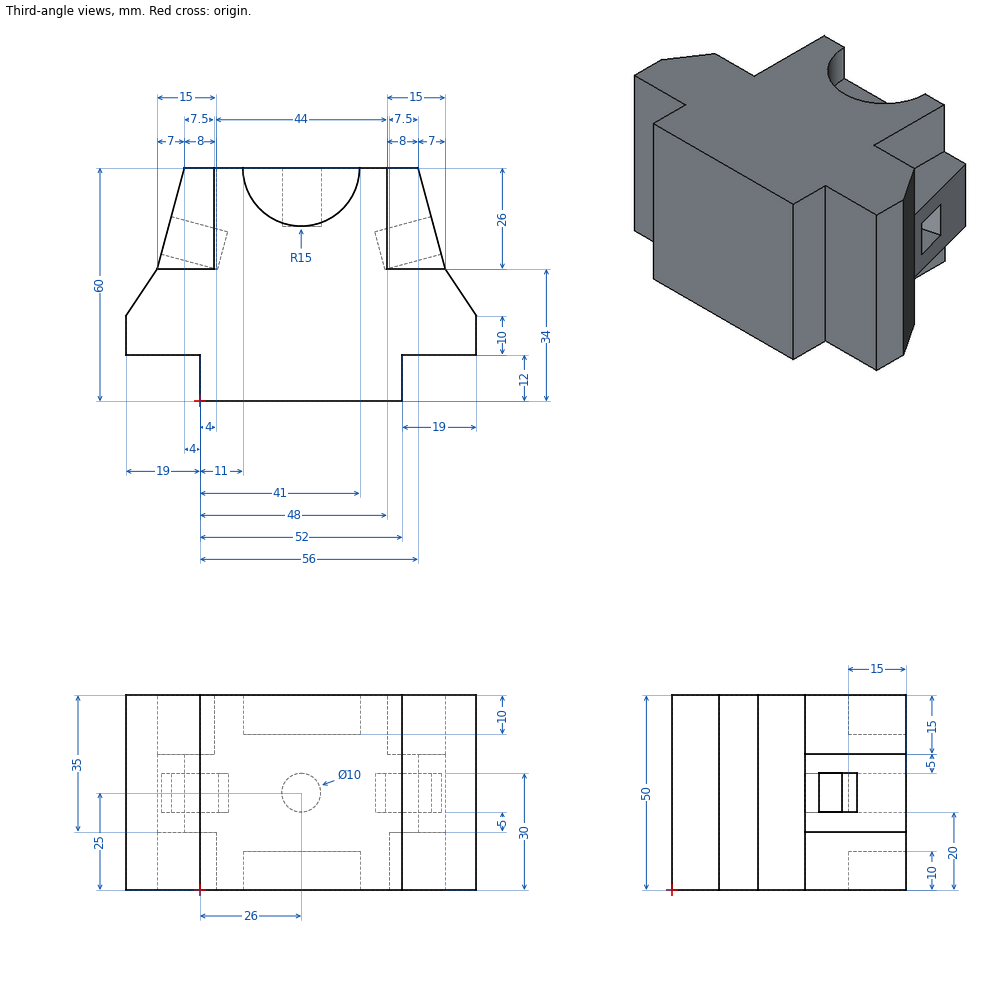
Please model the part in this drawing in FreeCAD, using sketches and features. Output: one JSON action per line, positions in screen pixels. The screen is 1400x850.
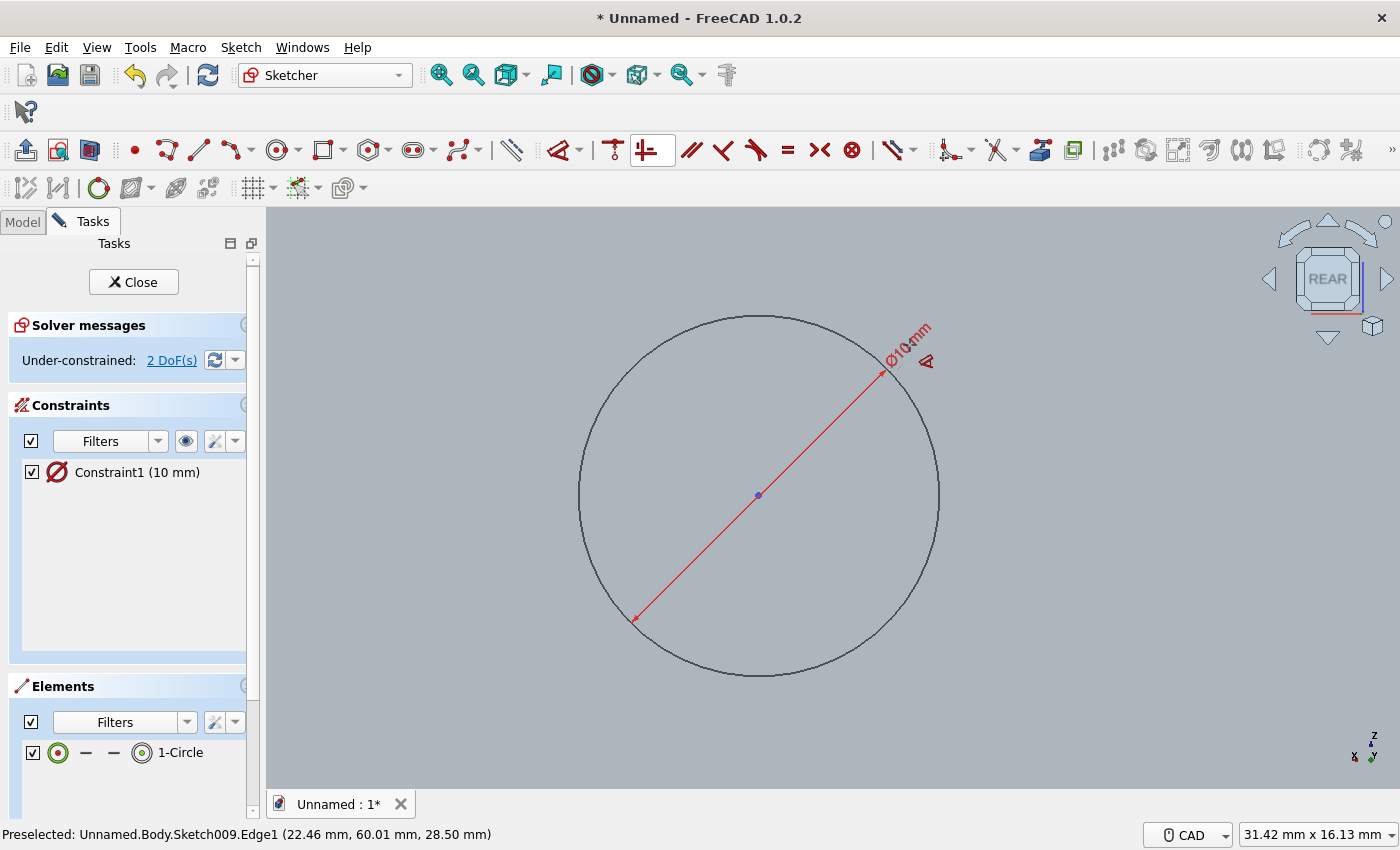
{"action": "left_click", "coordinate": [759, 496]}
{"action": "left_click", "coordinate": [997, 462]}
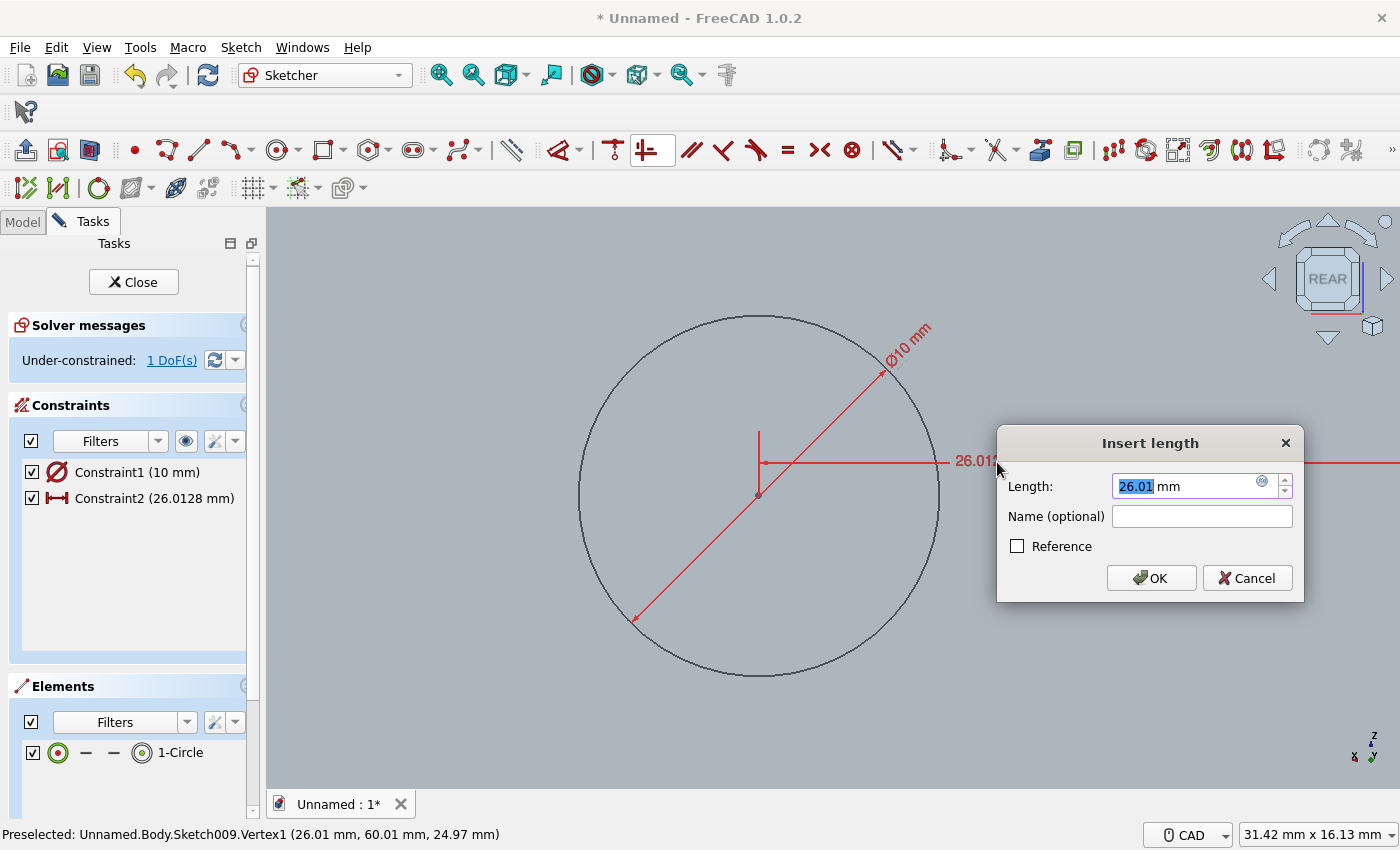
{"action": "type", "text": "26"}
{"action": "key", "text": "Return"}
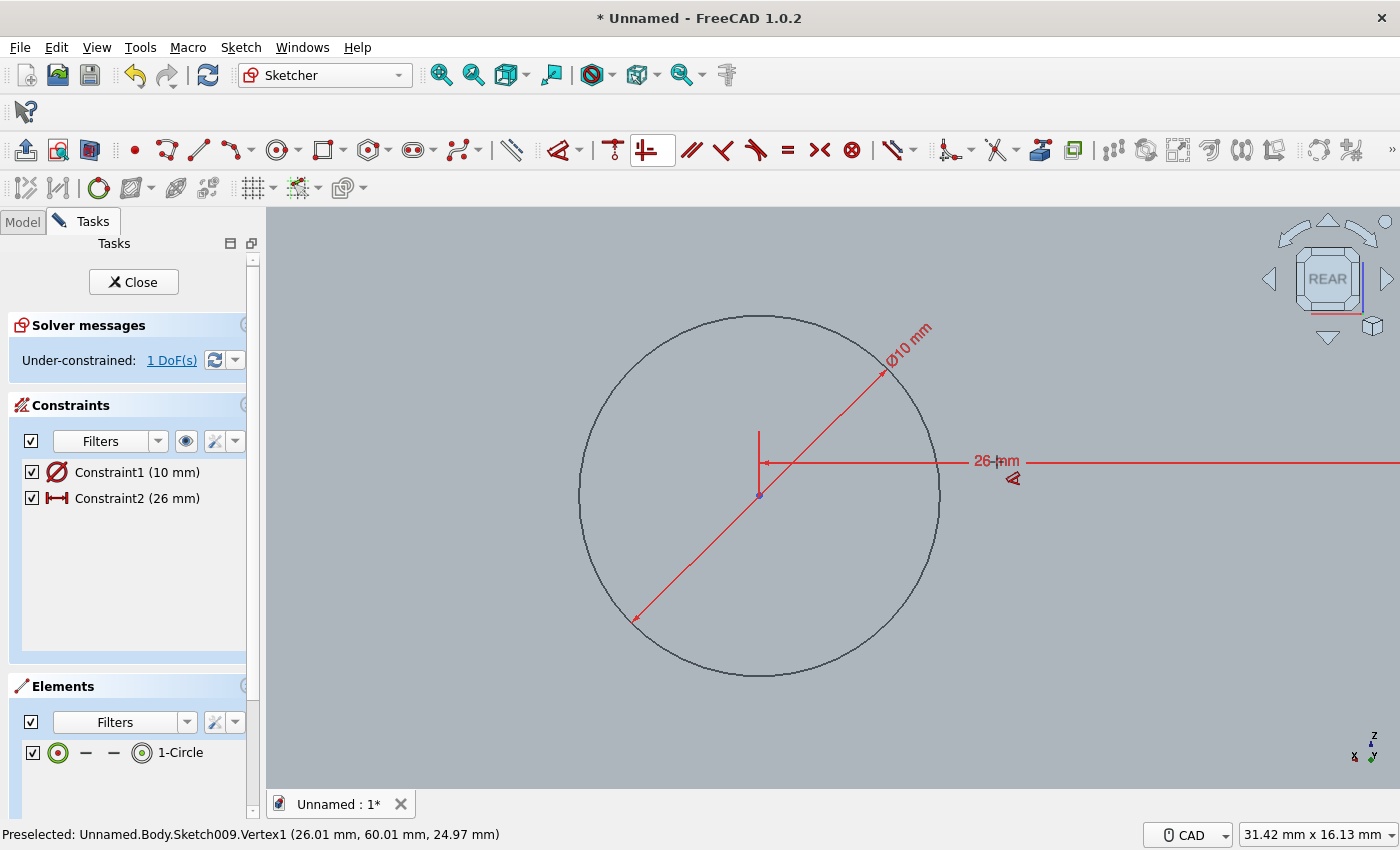
{"action": "left_click", "coordinate": [759, 496]}
{"action": "left_click", "coordinate": [725, 628]}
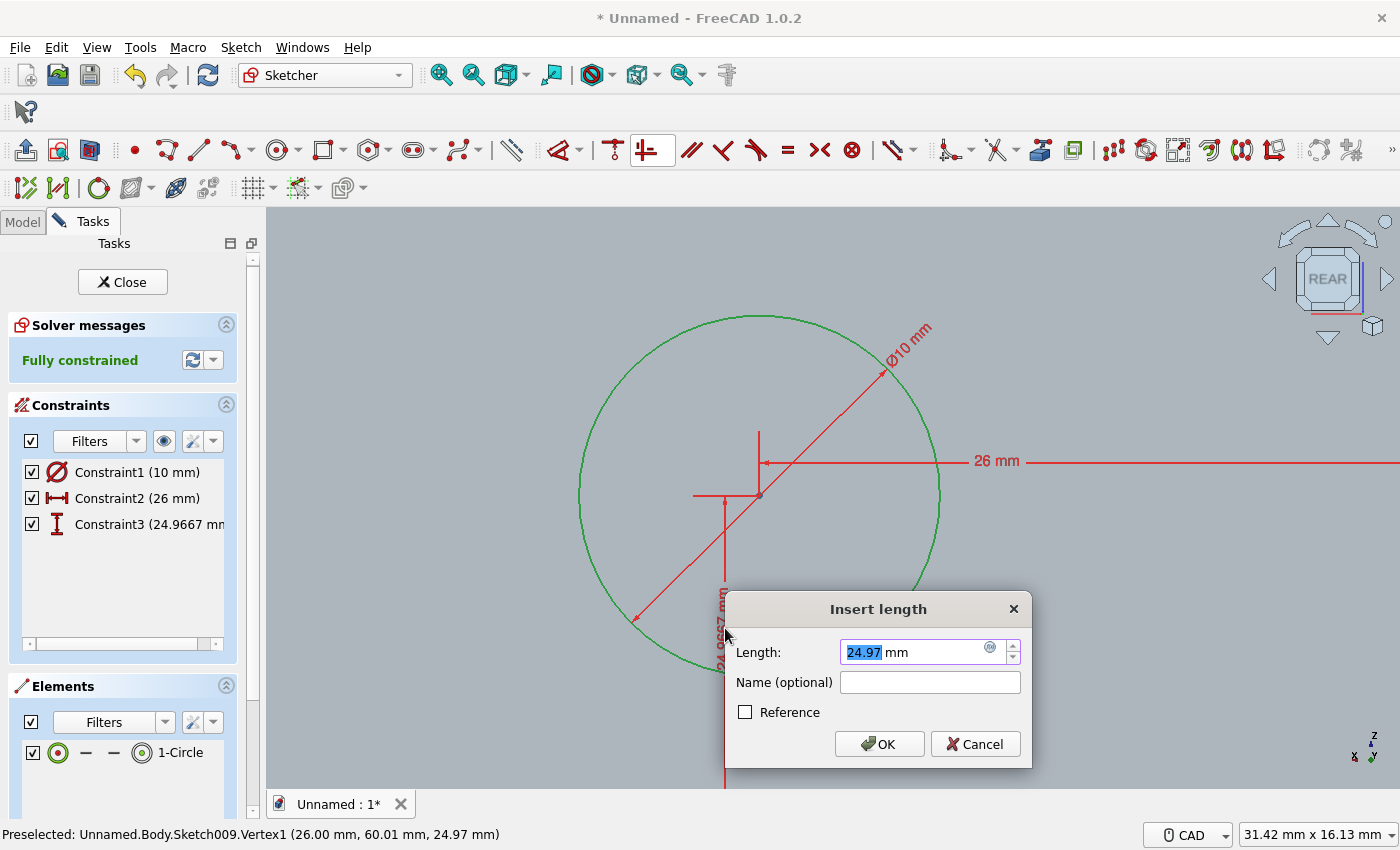
{"action": "type", "text": "25"}
{"action": "key", "text": "Return"}
{"action": "key", "text": "Escape"}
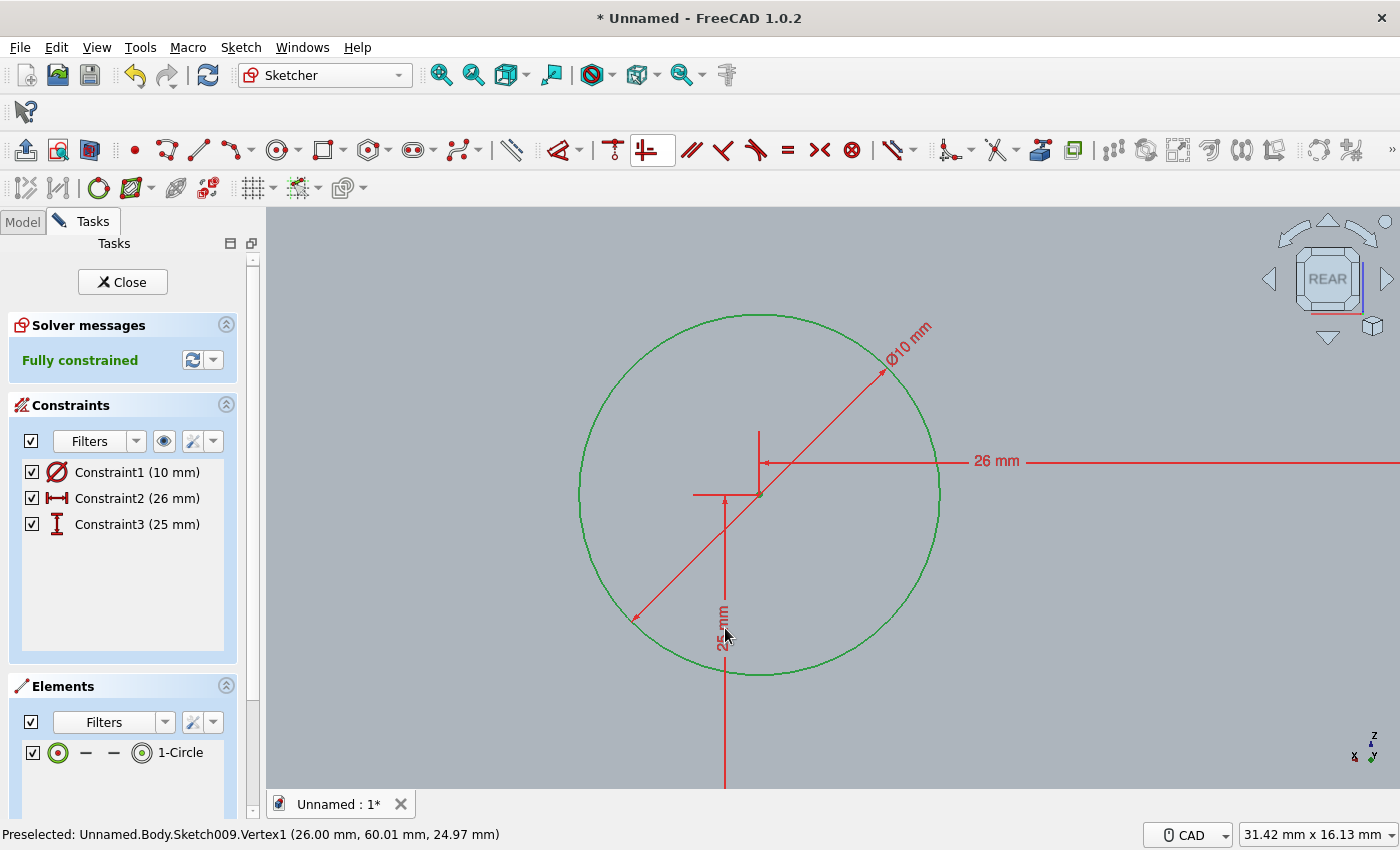
{"action": "left_click", "coordinate": [123, 282]}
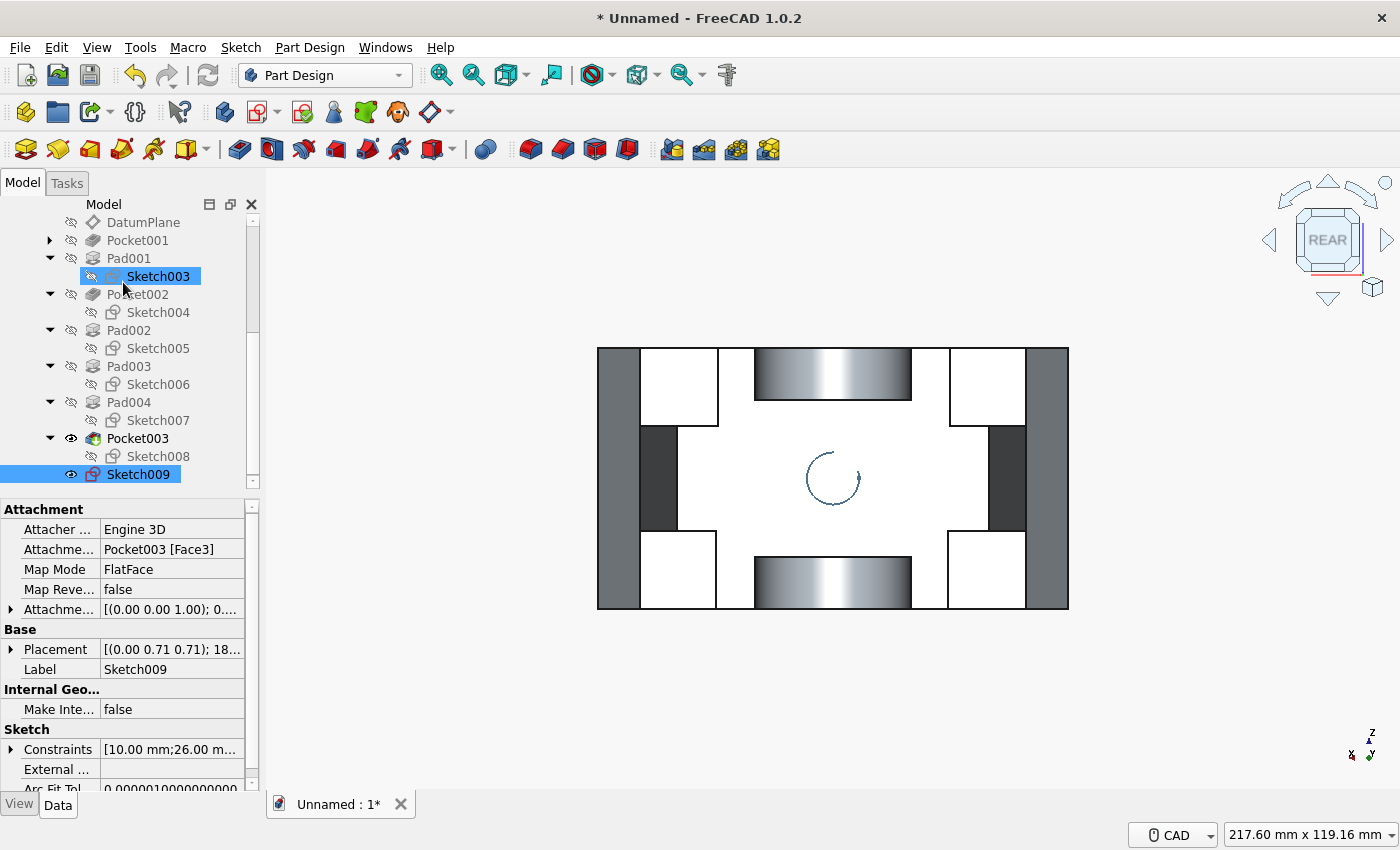
{"action": "left_click", "coordinate": [240, 150]}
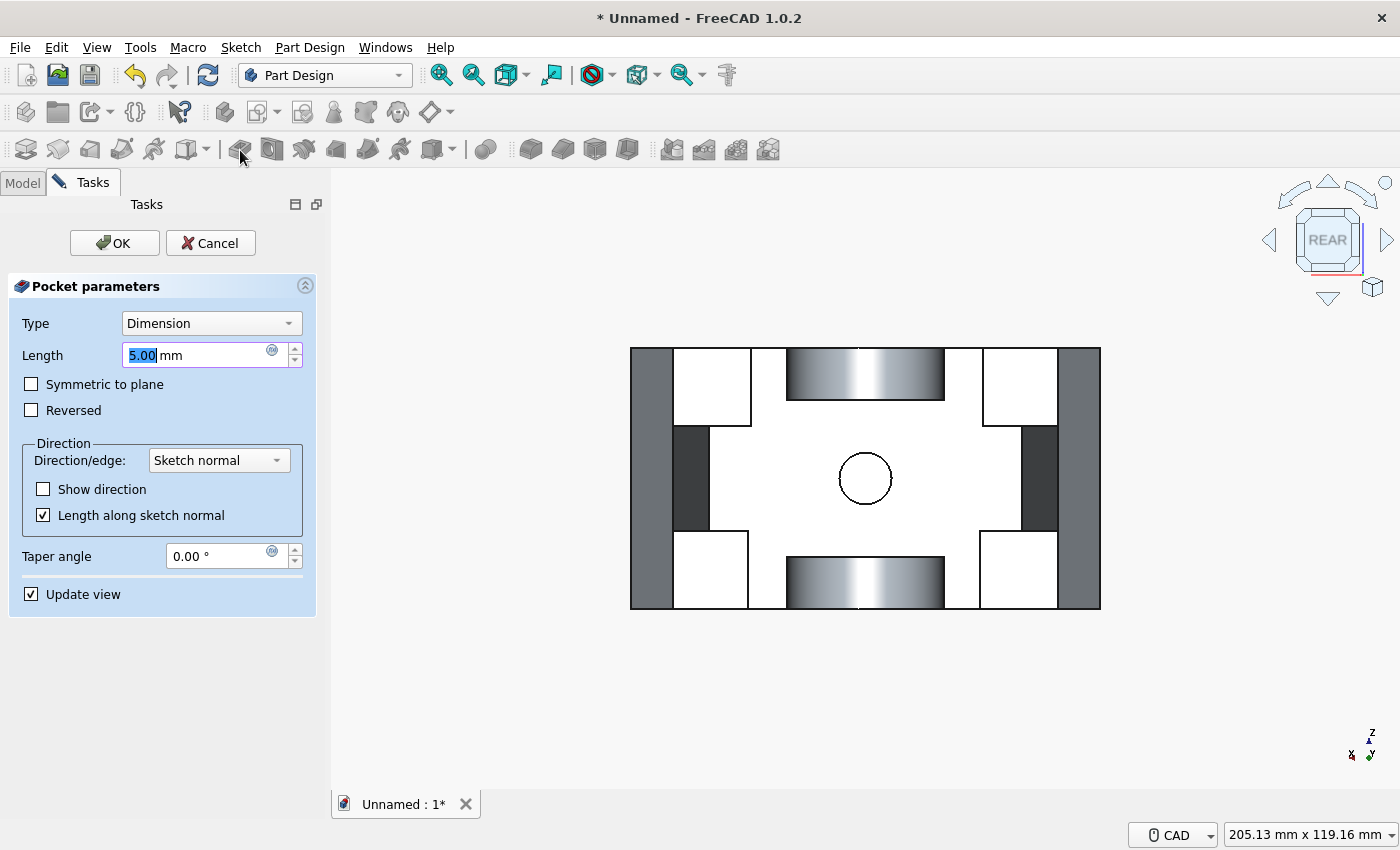
{"action": "type", "text": "15"}
{"action": "key", "text": "Tab"}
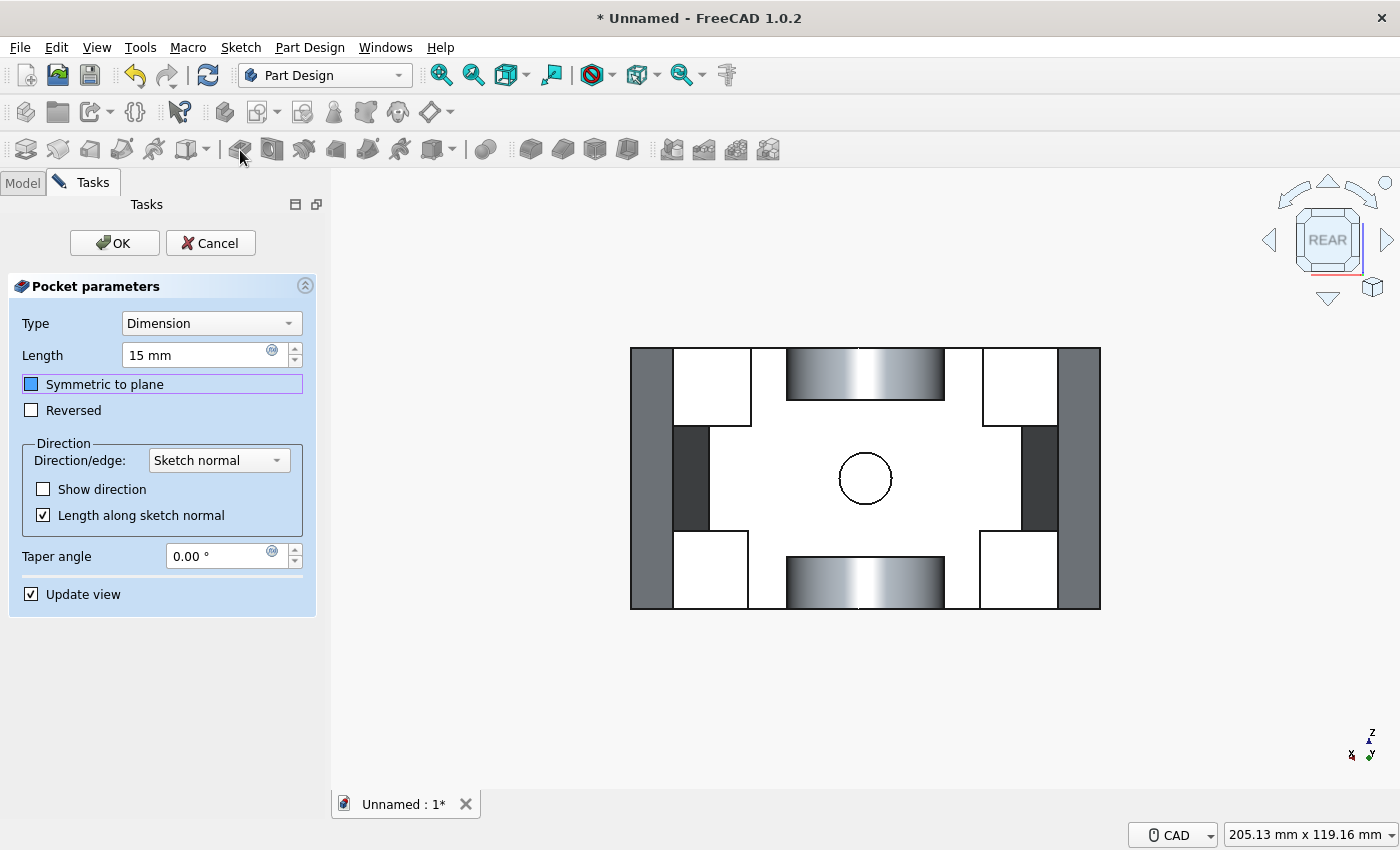
{"action": "left_click", "coordinate": [115, 243]}